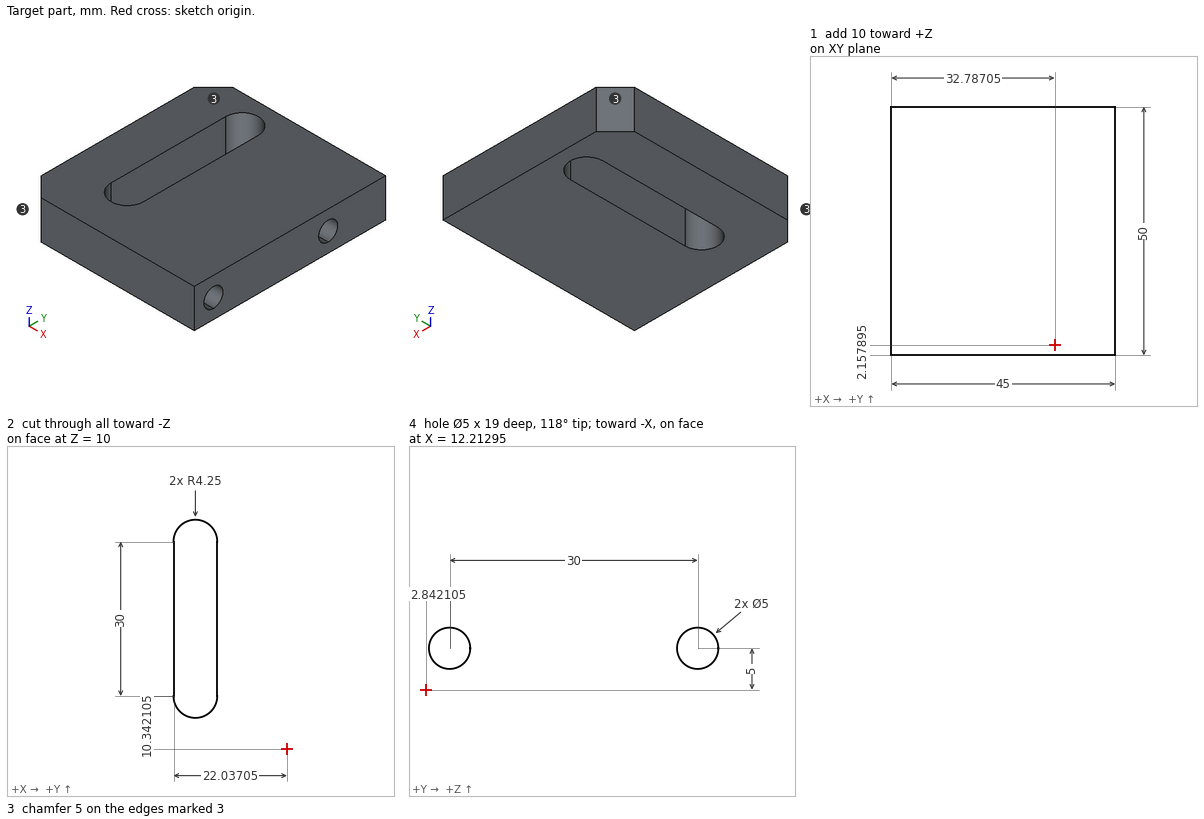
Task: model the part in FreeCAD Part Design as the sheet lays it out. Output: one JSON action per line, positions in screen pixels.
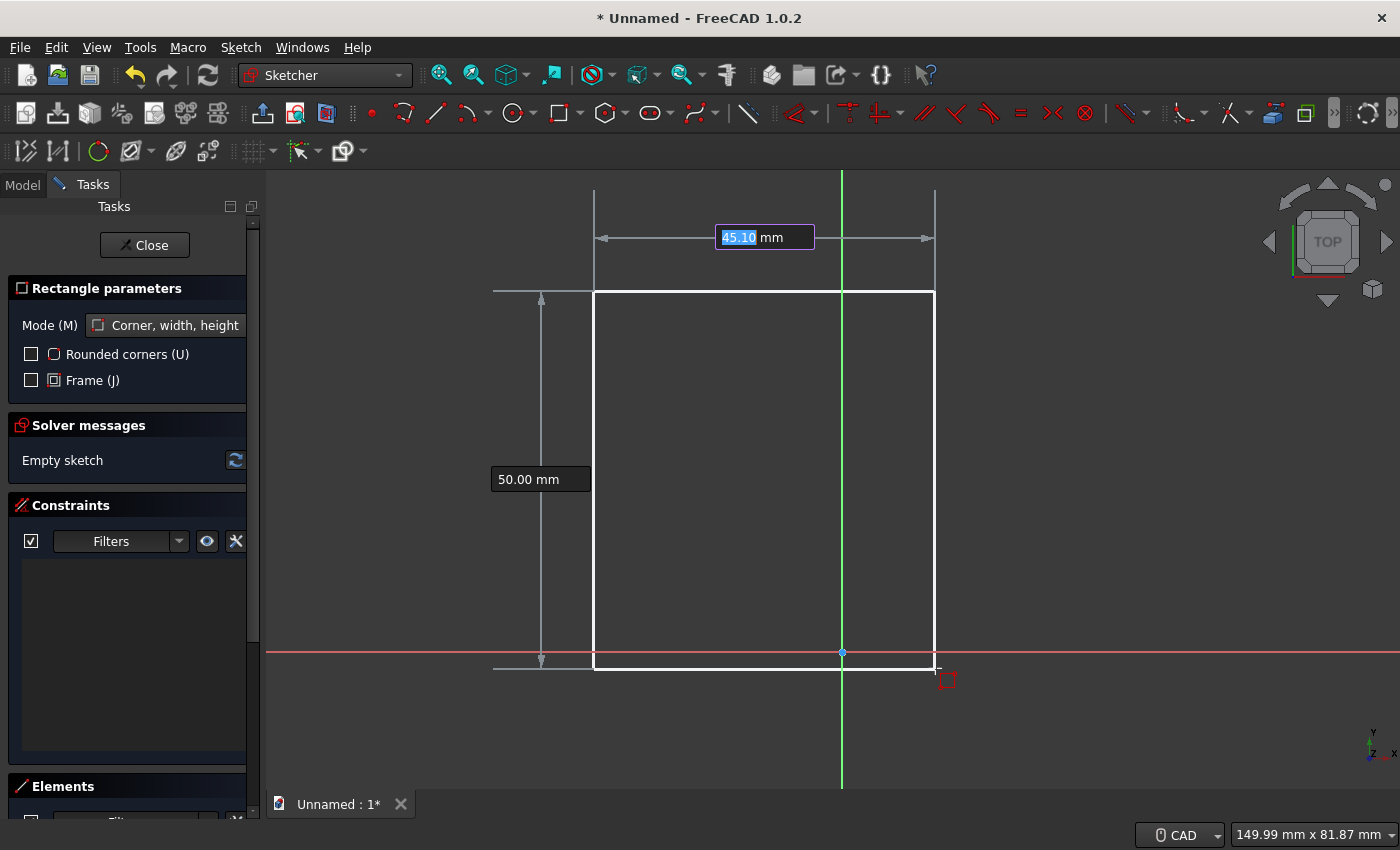
{"action": "type", "text": "45"}
{"action": "key", "text": "Tab"}
{"action": "type", "text": "50"}
{"action": "key", "text": "Return"}
{"action": "key", "text": "Escape"}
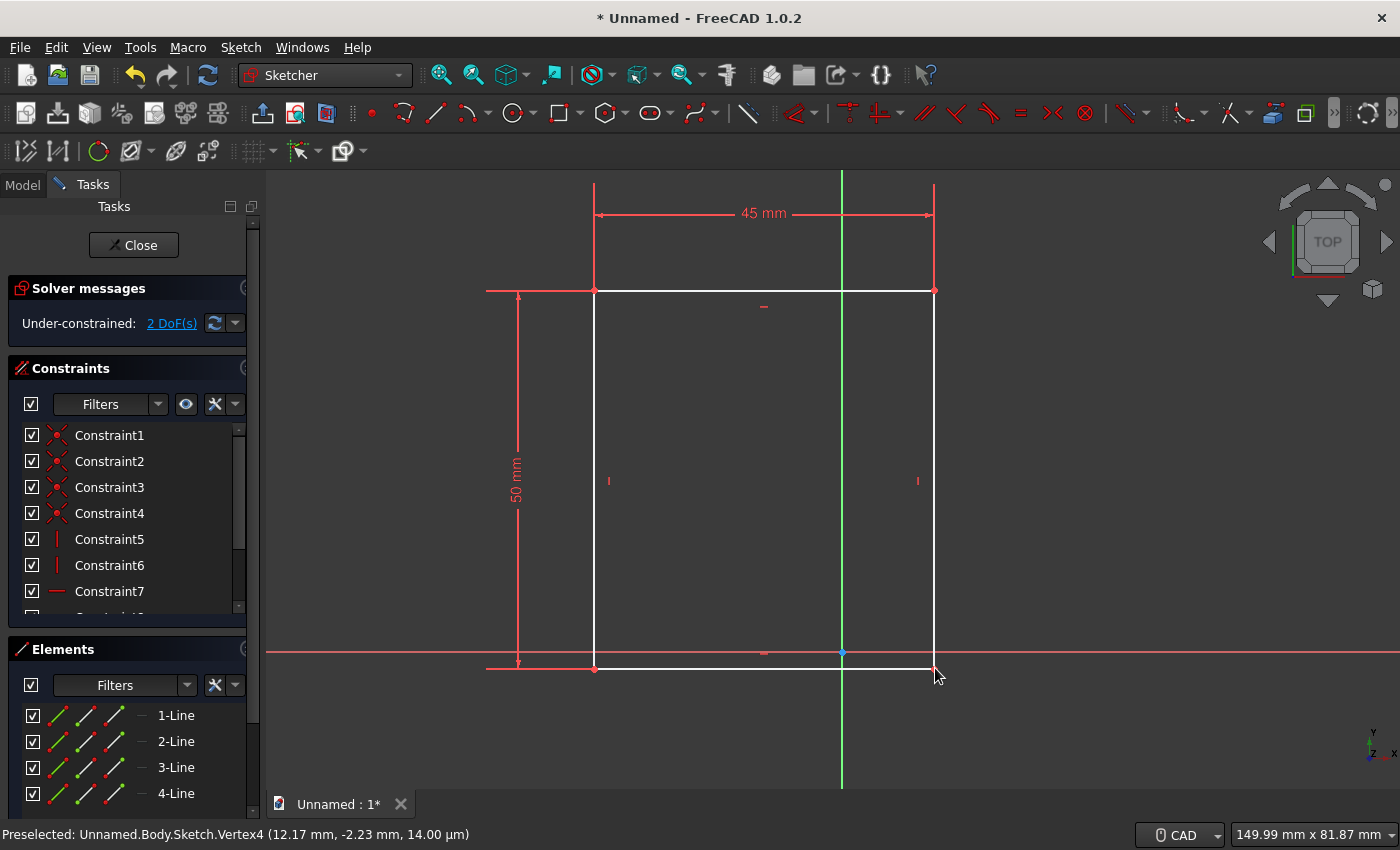
{"action": "left_click", "coordinate": [794, 114]}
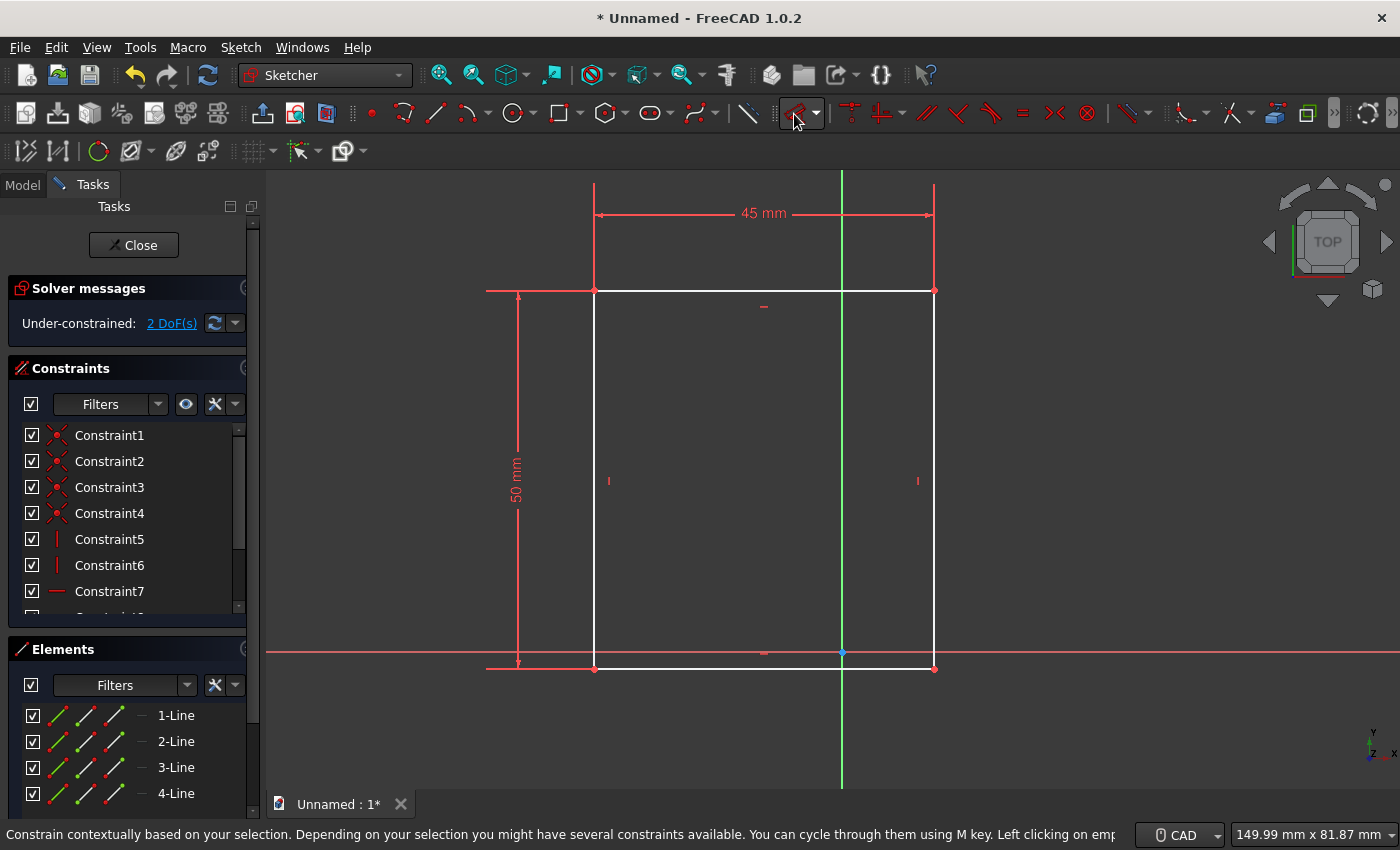
{"action": "left_click", "coordinate": [594, 291]}
{"action": "left_click", "coordinate": [718, 257]}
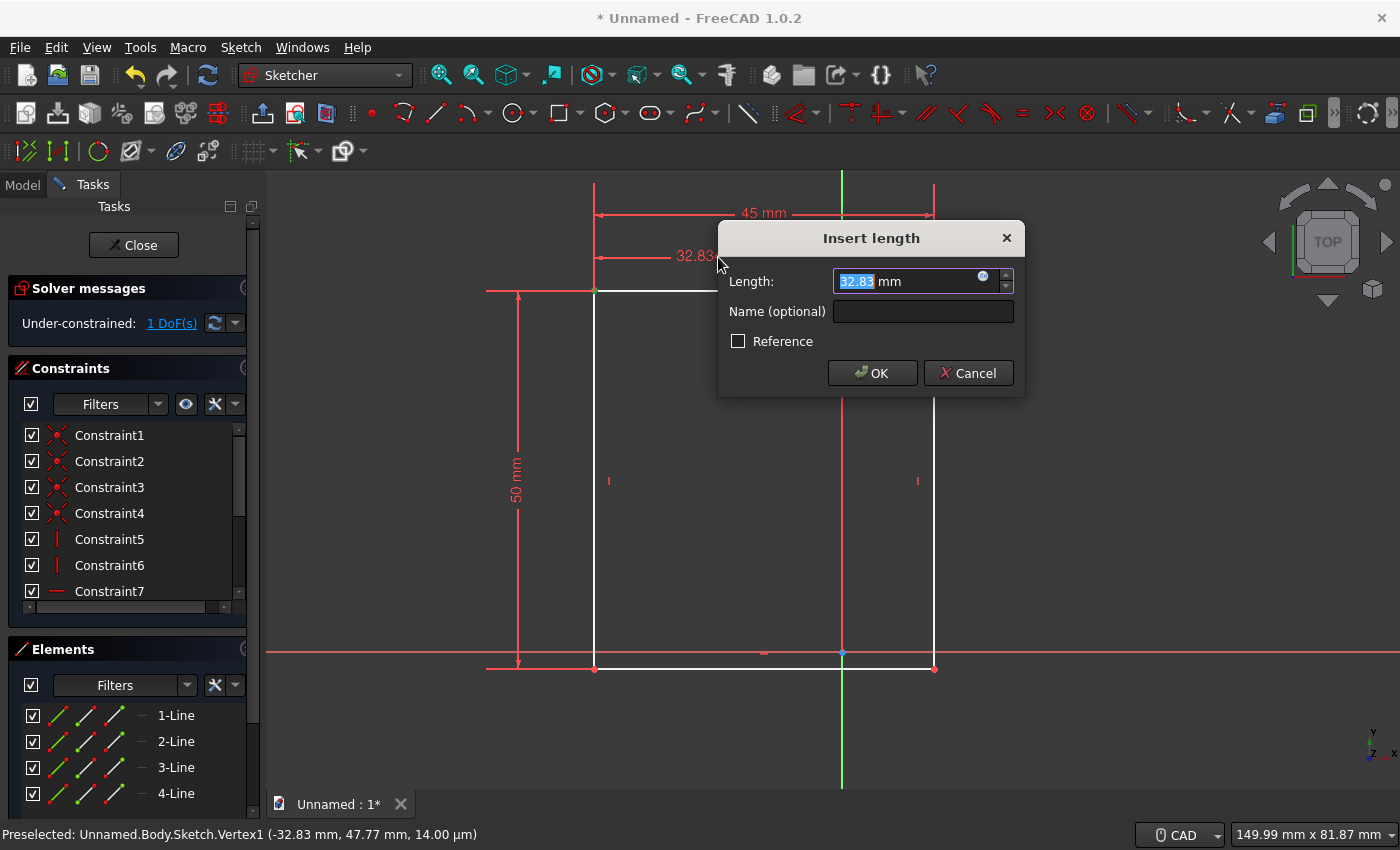
{"action": "type", "text": "32.78705"}
{"action": "key", "text": "Return"}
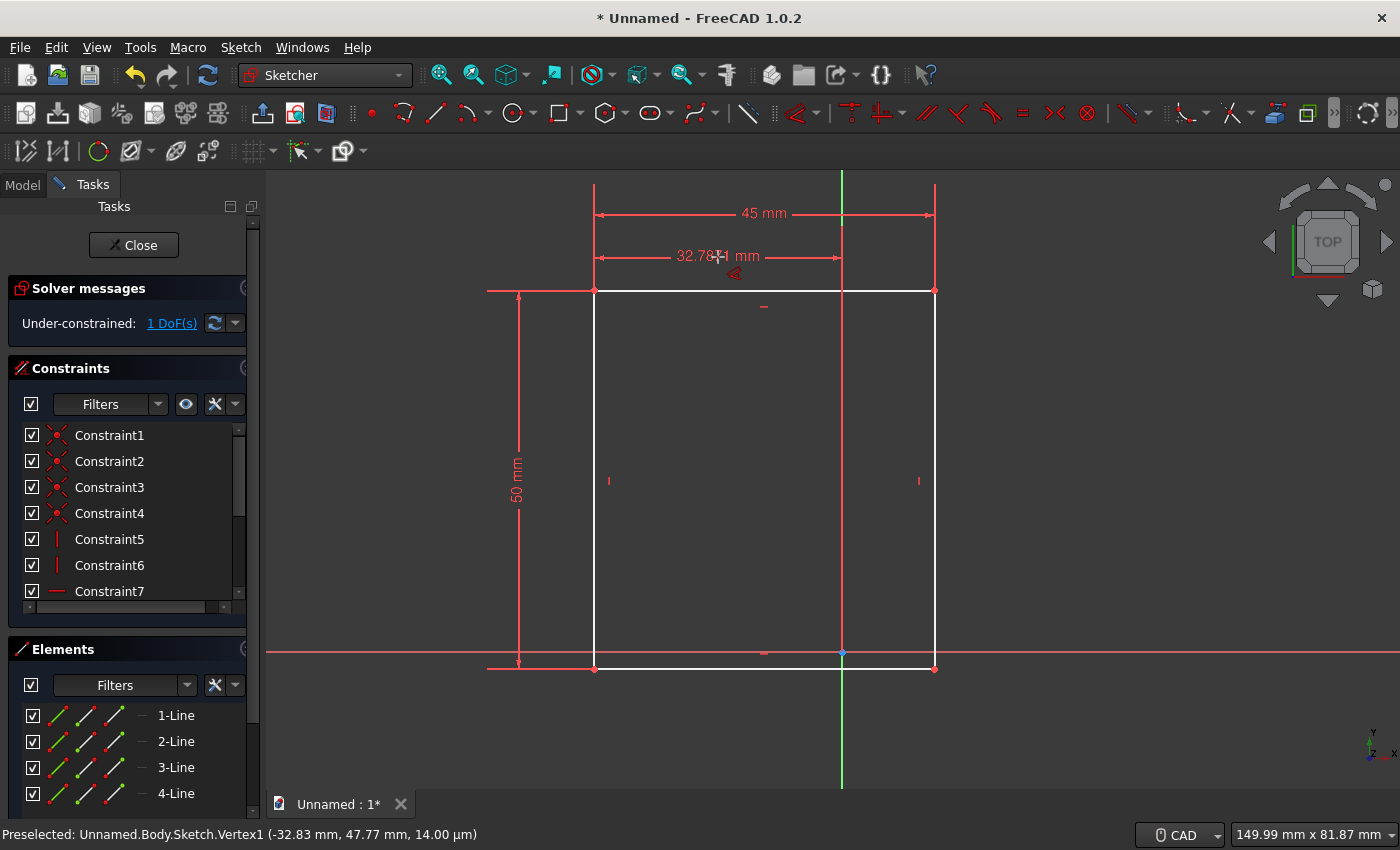
{"action": "scroll", "coordinate": [594, 669], "scroll_direction": "up", "scroll_amount": 5}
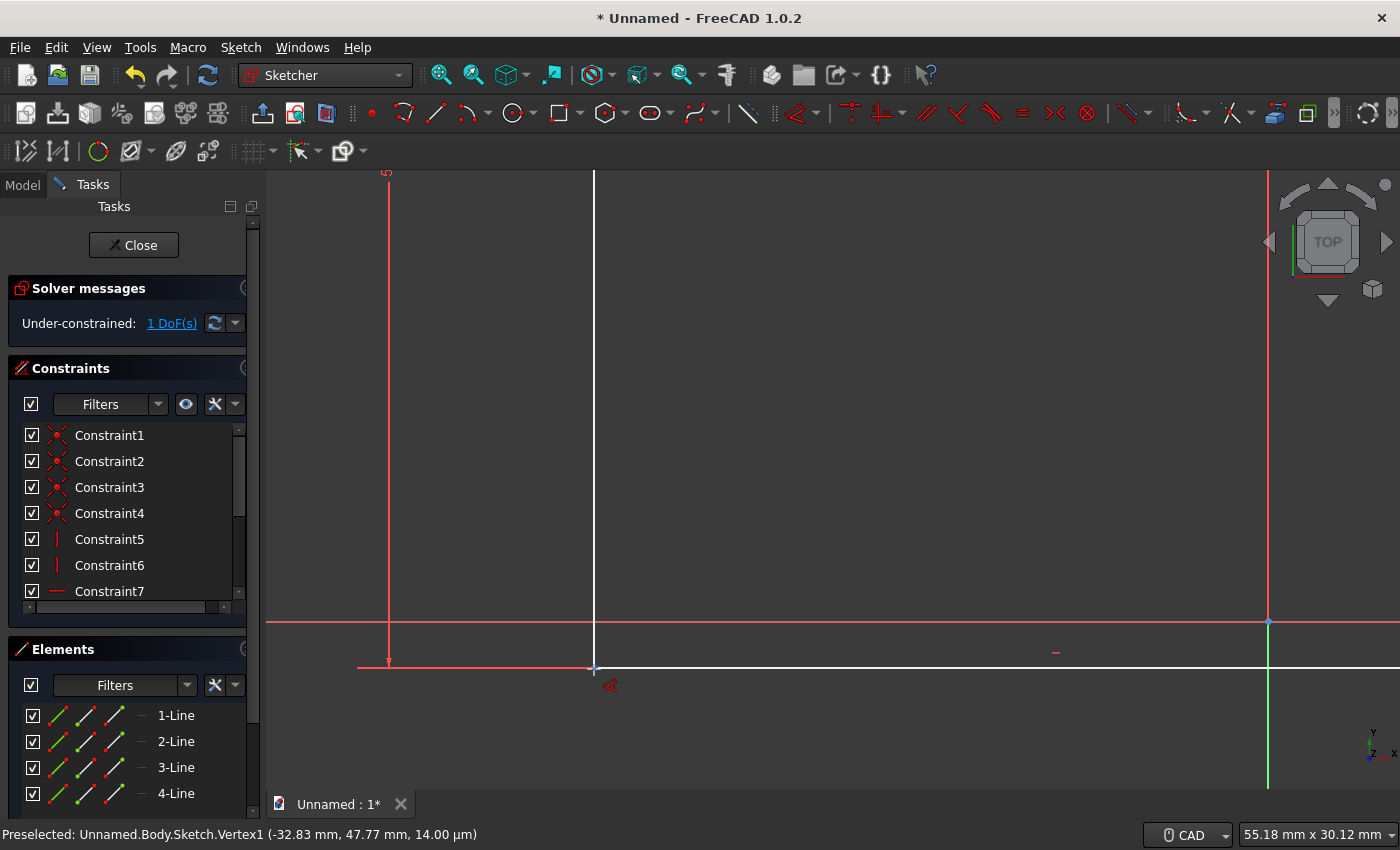
{"action": "left_click", "coordinate": [594, 668]}
{"action": "left_click", "coordinate": [560, 645]}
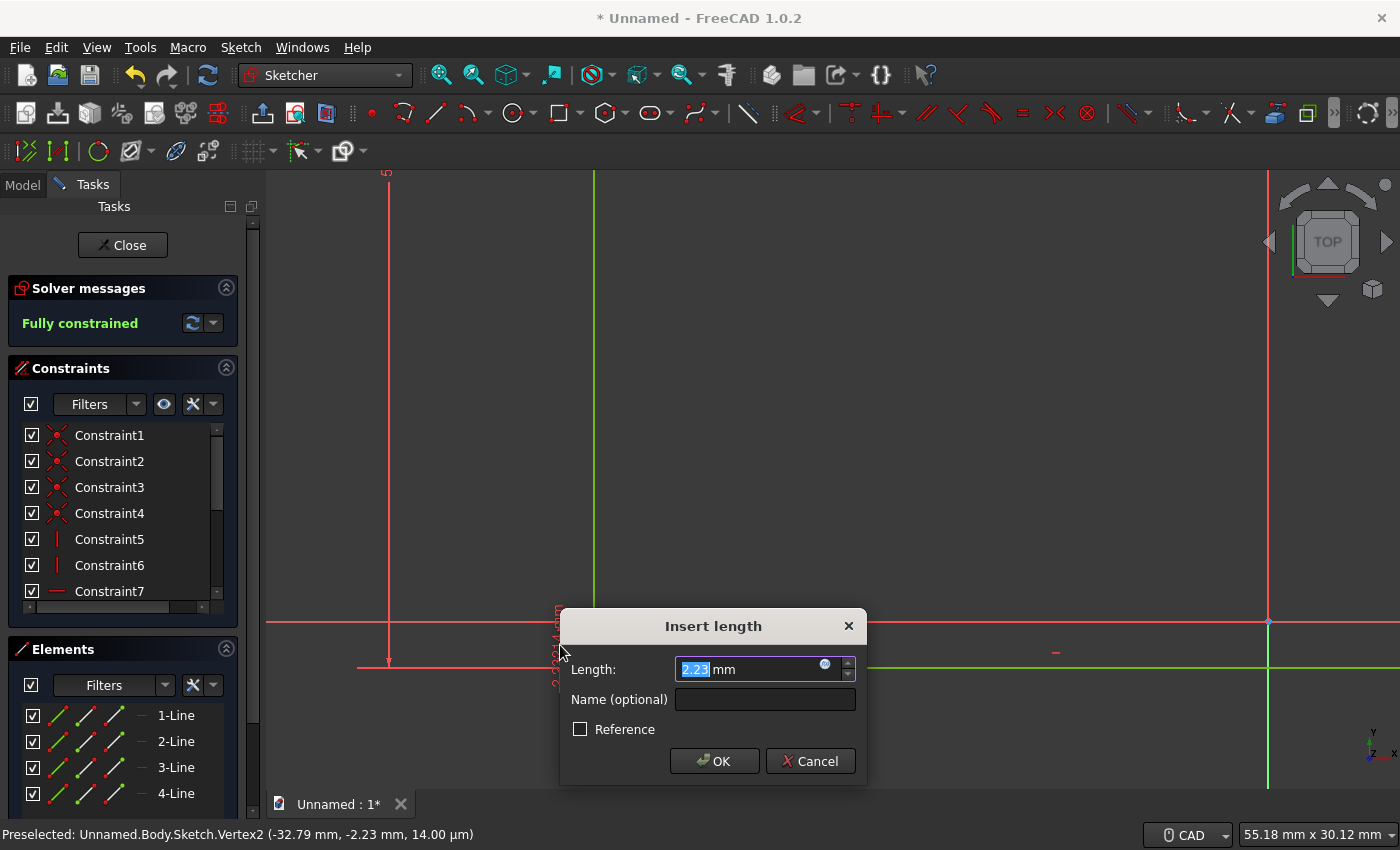
{"action": "type", "text": "2.157895"}
{"action": "key", "text": "Return"}
{"action": "key", "text": "Escape"}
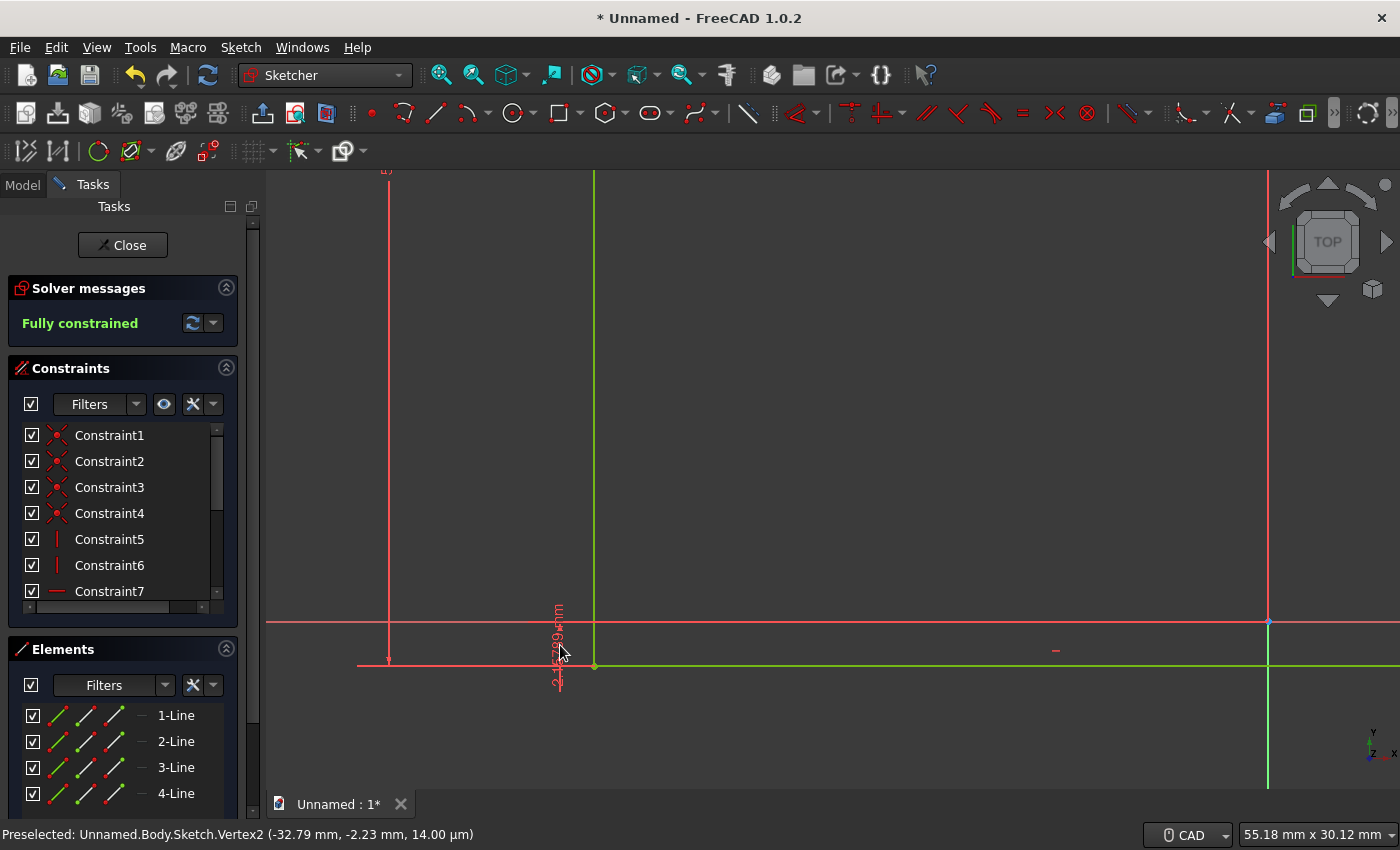
{"action": "left_click", "coordinate": [123, 245]}